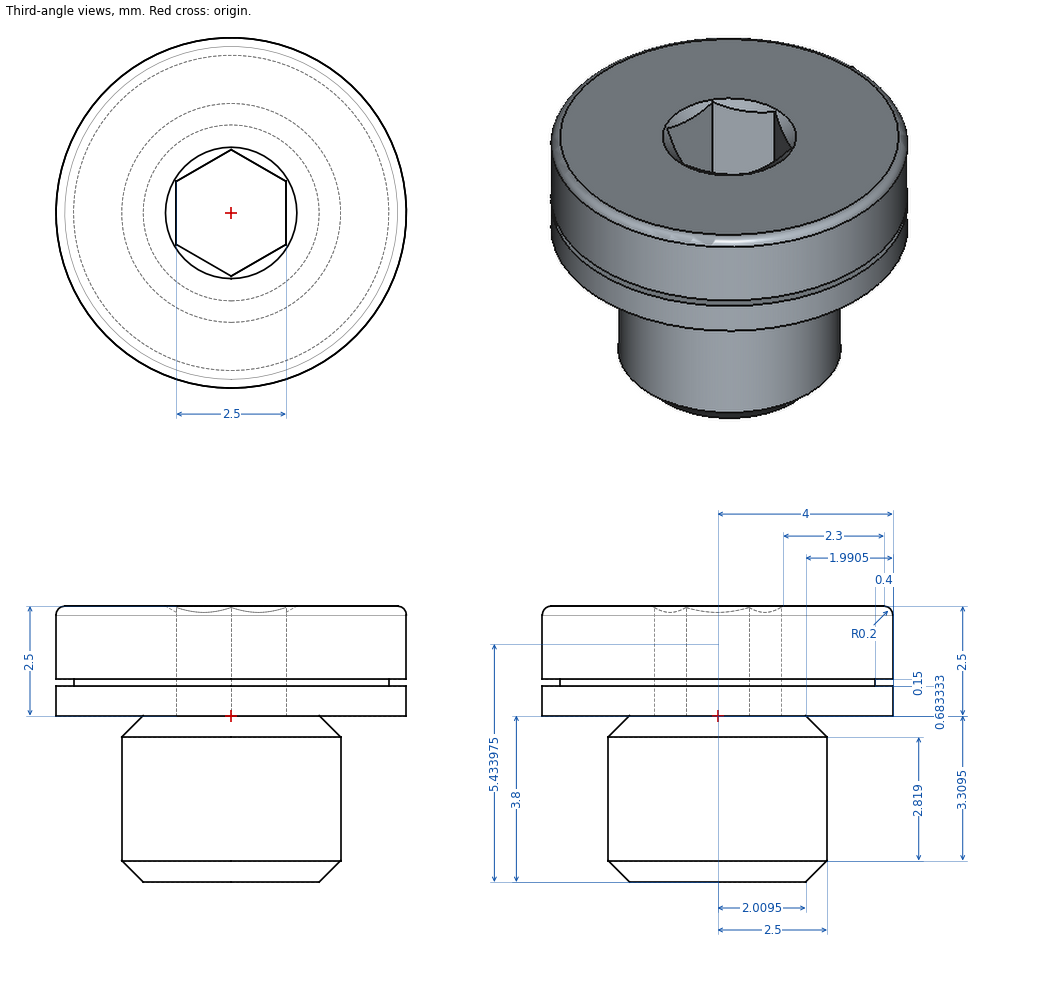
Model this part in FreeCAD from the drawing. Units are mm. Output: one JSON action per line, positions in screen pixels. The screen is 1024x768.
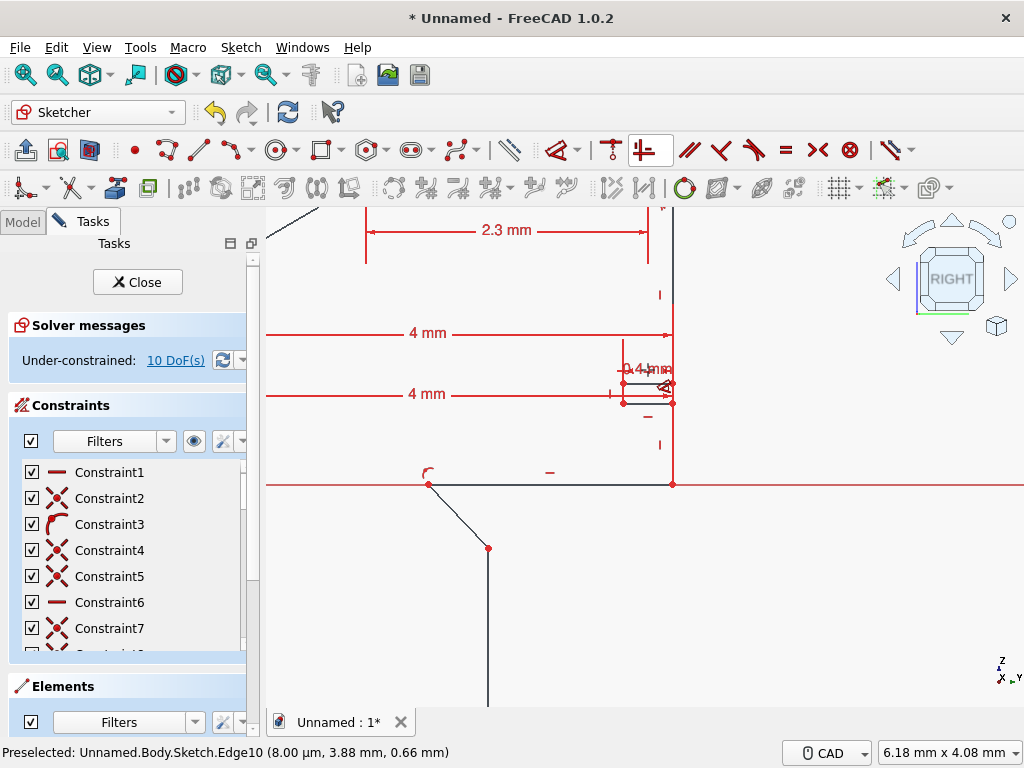
{"action": "scroll", "coordinate": [623, 394], "scroll_direction": "up", "scroll_amount": 4}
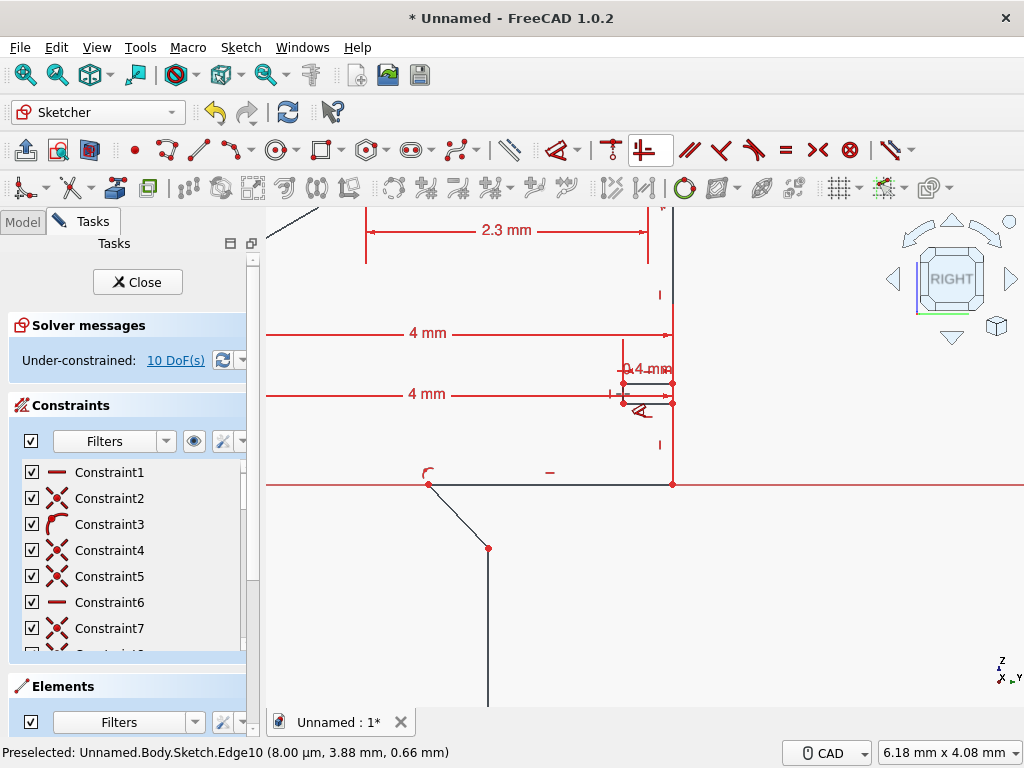
{"action": "left_click", "coordinate": [623, 393]}
{"action": "left_click", "coordinate": [657, 393]}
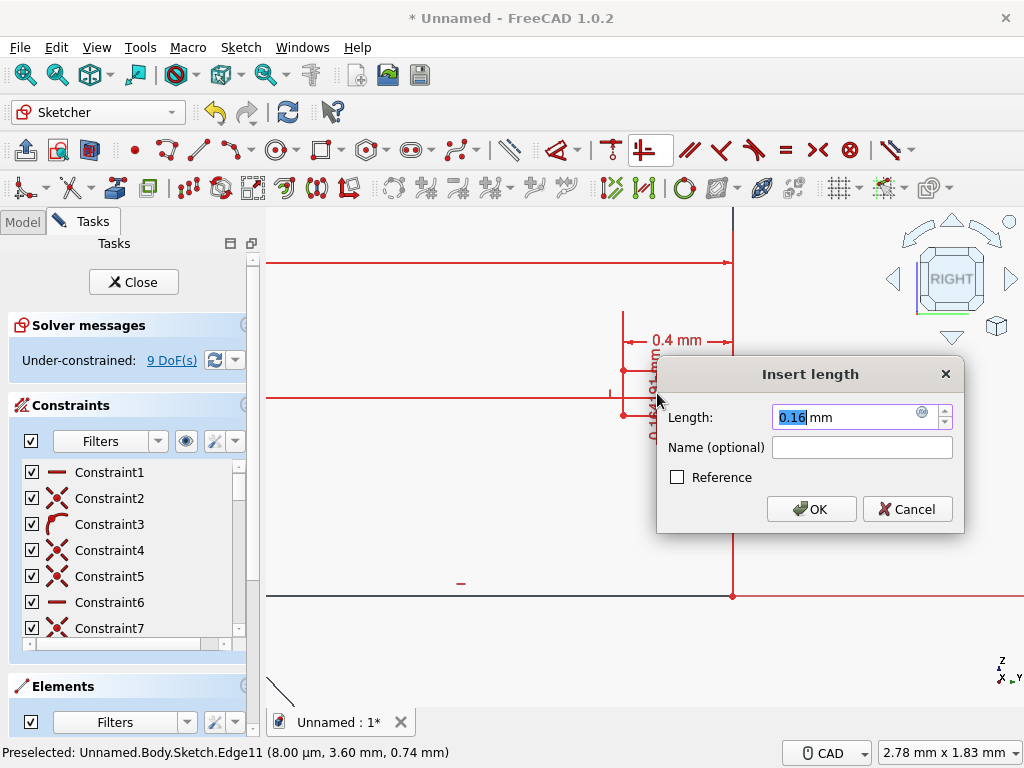
{"action": "type", "text": "0.15"}
{"action": "key", "text": "Return"}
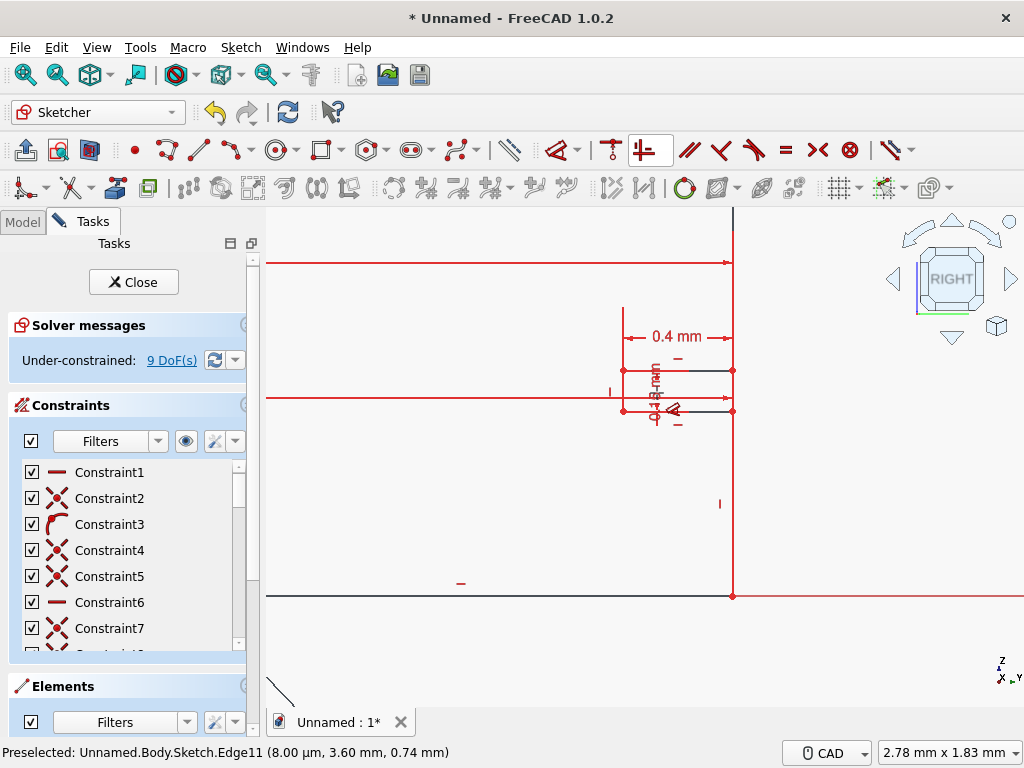
{"action": "scroll", "coordinate": [654, 394], "scroll_direction": "down", "scroll_amount": 9}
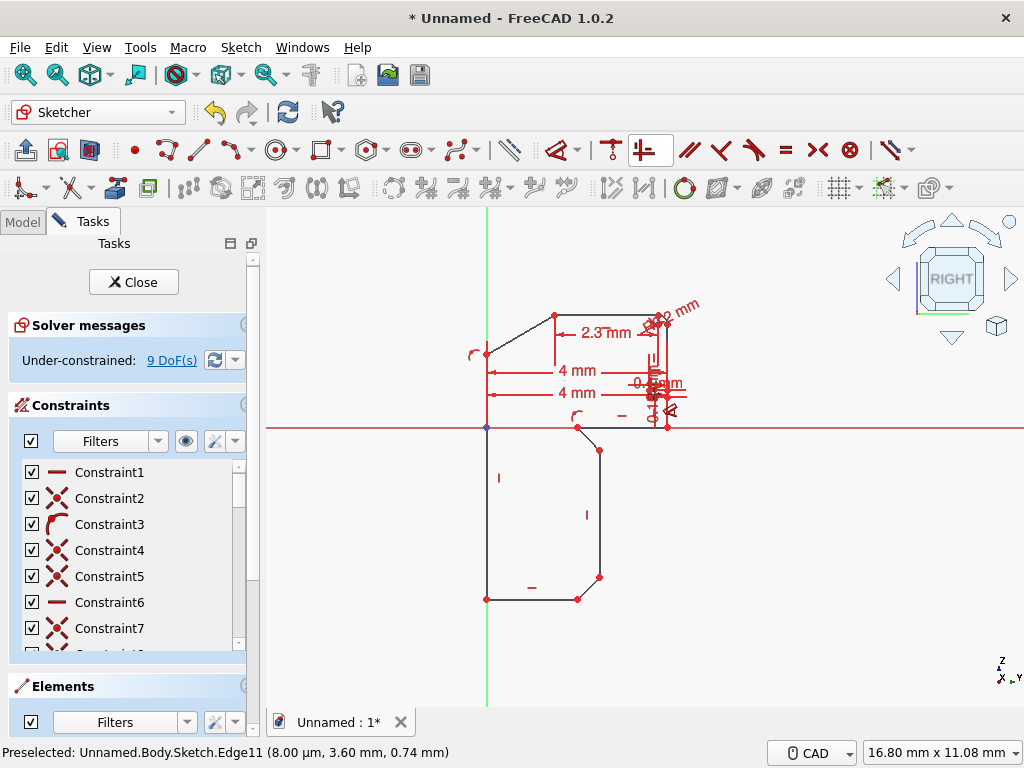
{"action": "scroll", "coordinate": [658, 315], "scroll_direction": "up", "scroll_amount": 2}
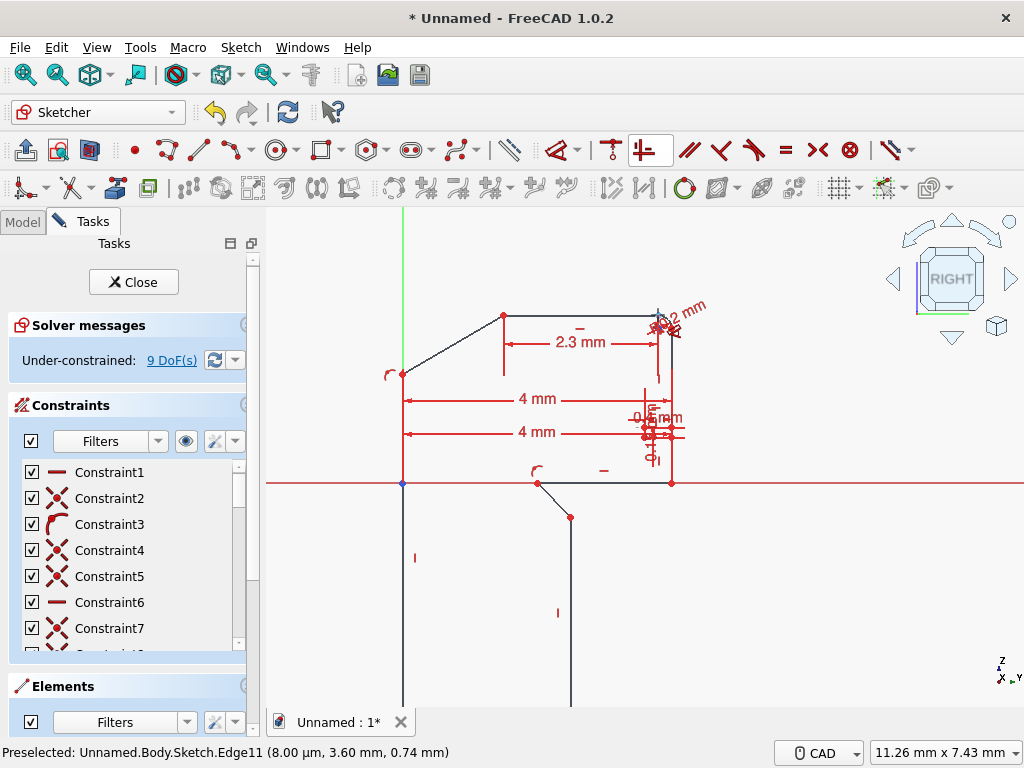
{"action": "left_click", "coordinate": [658, 316]}
{"action": "left_click", "coordinate": [369, 399]}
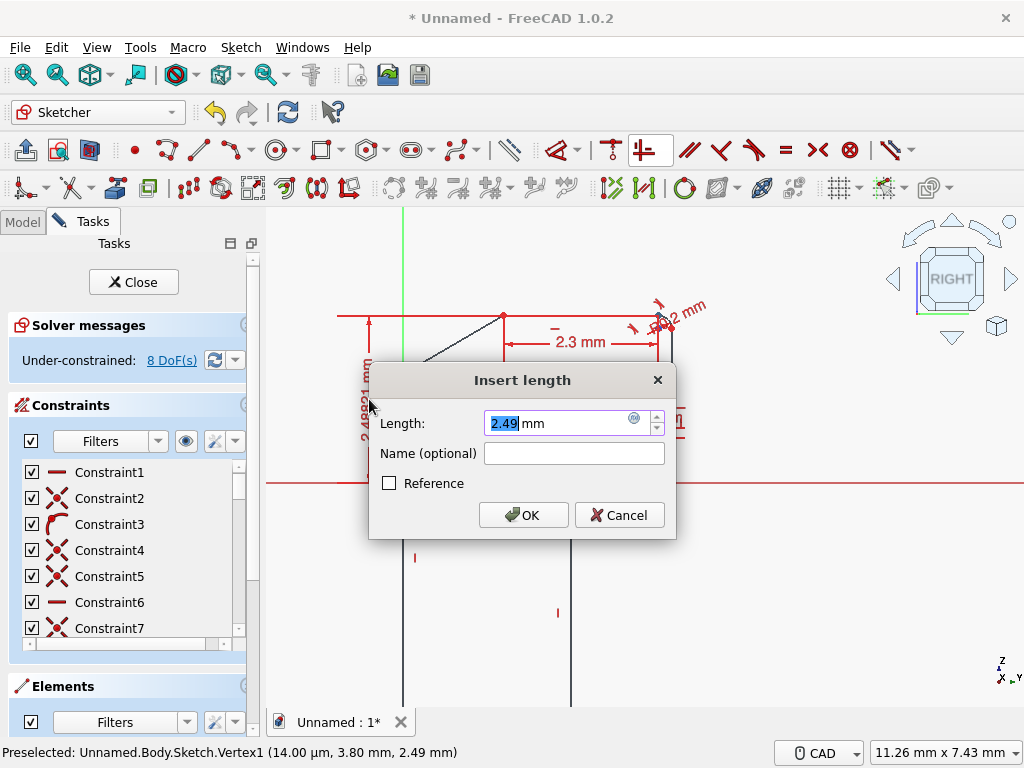
{"action": "type", "text": "2.5"}
{"action": "key", "text": "Return"}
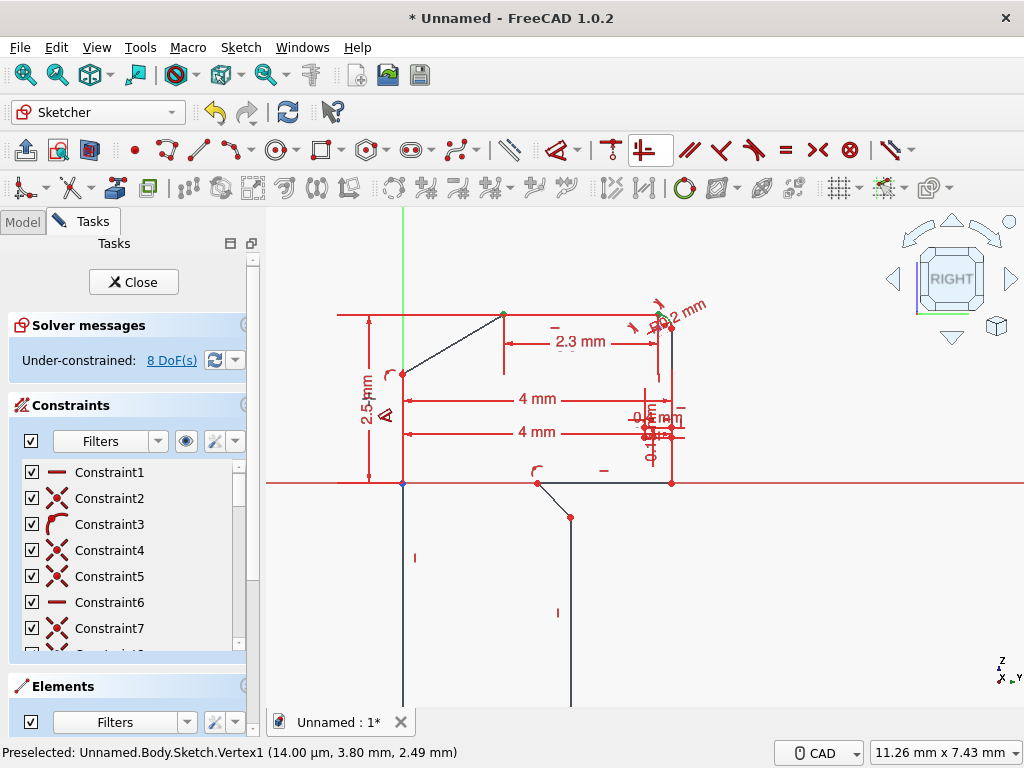
{"action": "scroll", "coordinate": [656, 315], "scroll_direction": "down", "scroll_amount": 2}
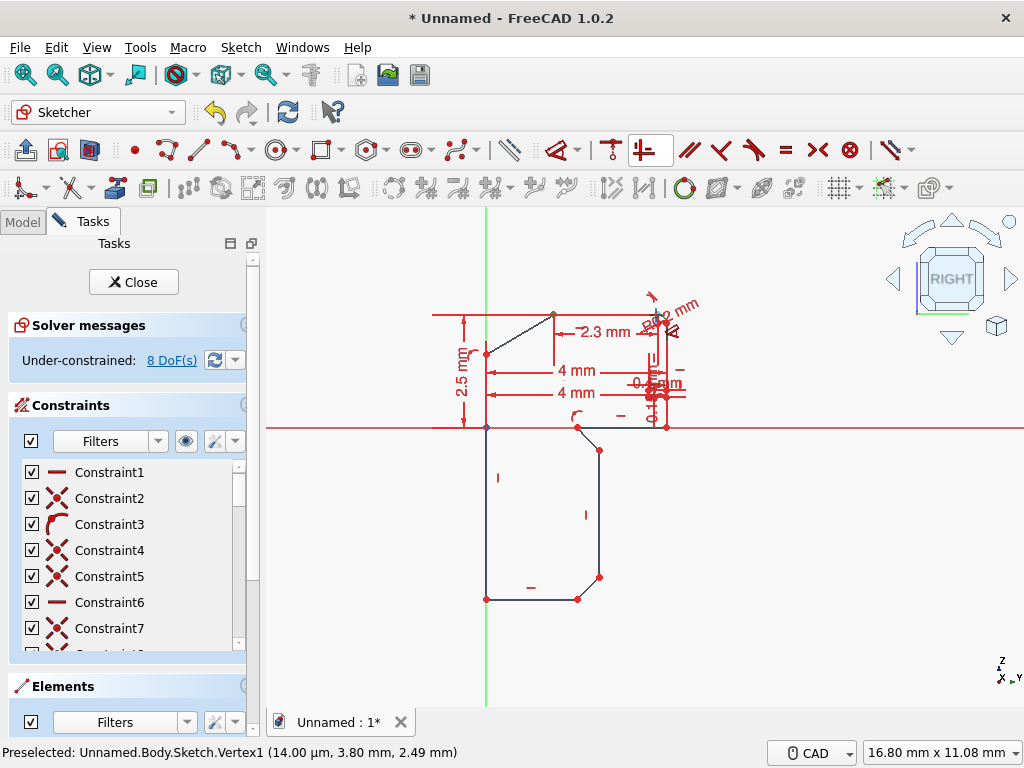
{"action": "left_click", "coordinate": [486, 600]}
{"action": "left_click", "coordinate": [452, 514]}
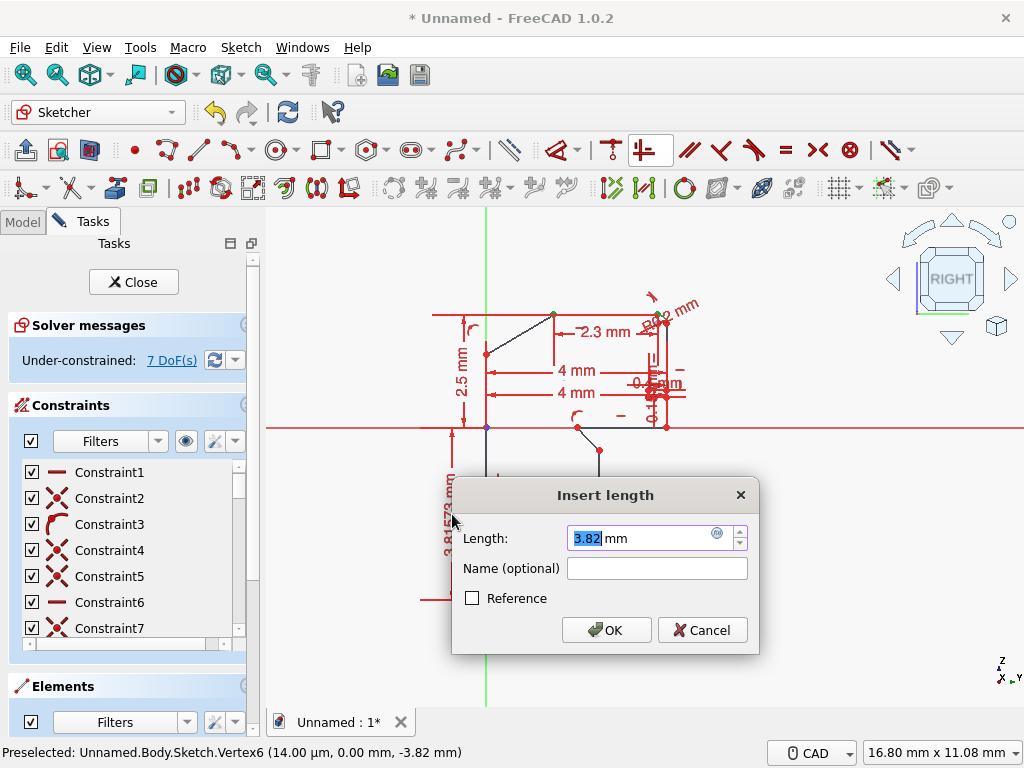
{"action": "type", "text": "3.8"}
{"action": "key", "text": "Return"}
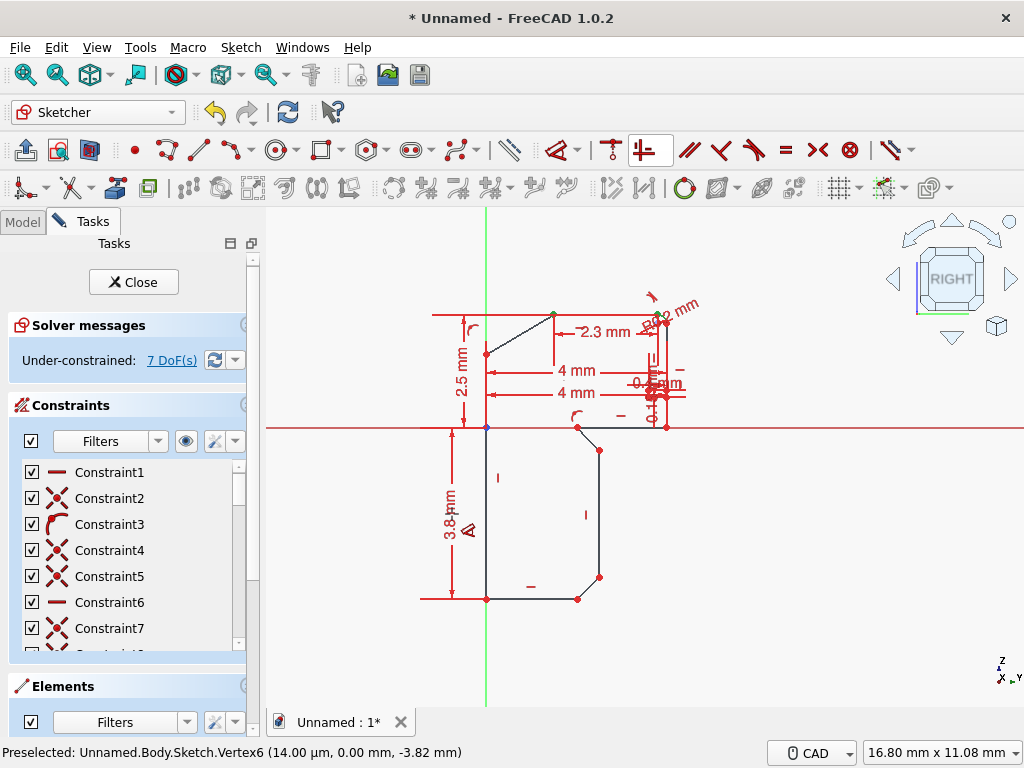
{"action": "left_click", "coordinate": [599, 578]}
{"action": "left_click", "coordinate": [582, 612]}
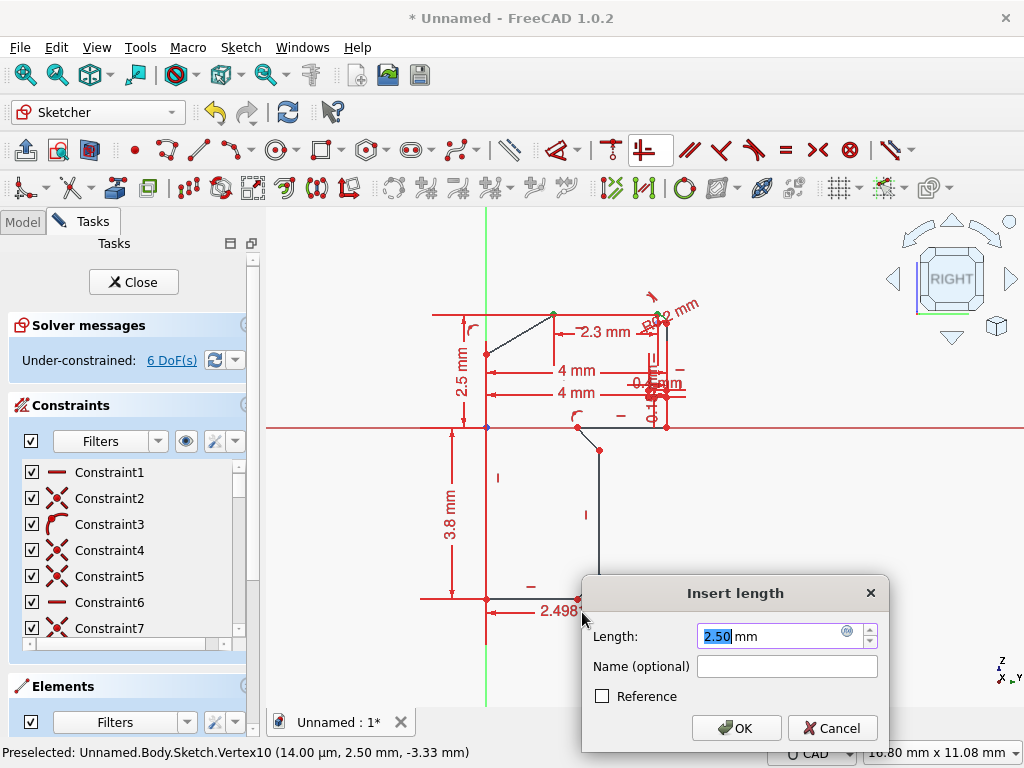
{"action": "type", "text": "2.5"}
{"action": "key", "text": "Return"}